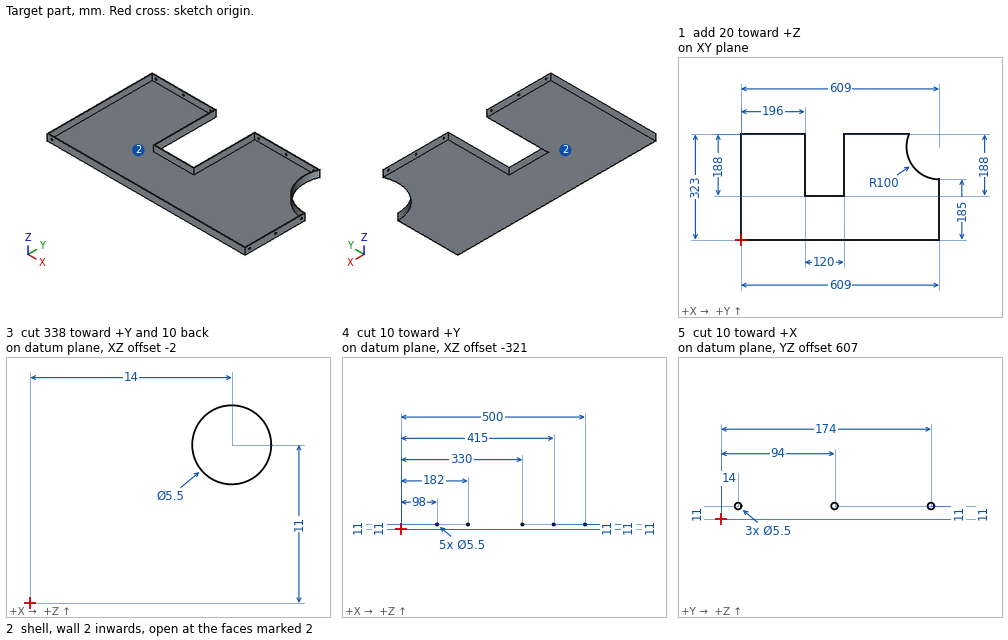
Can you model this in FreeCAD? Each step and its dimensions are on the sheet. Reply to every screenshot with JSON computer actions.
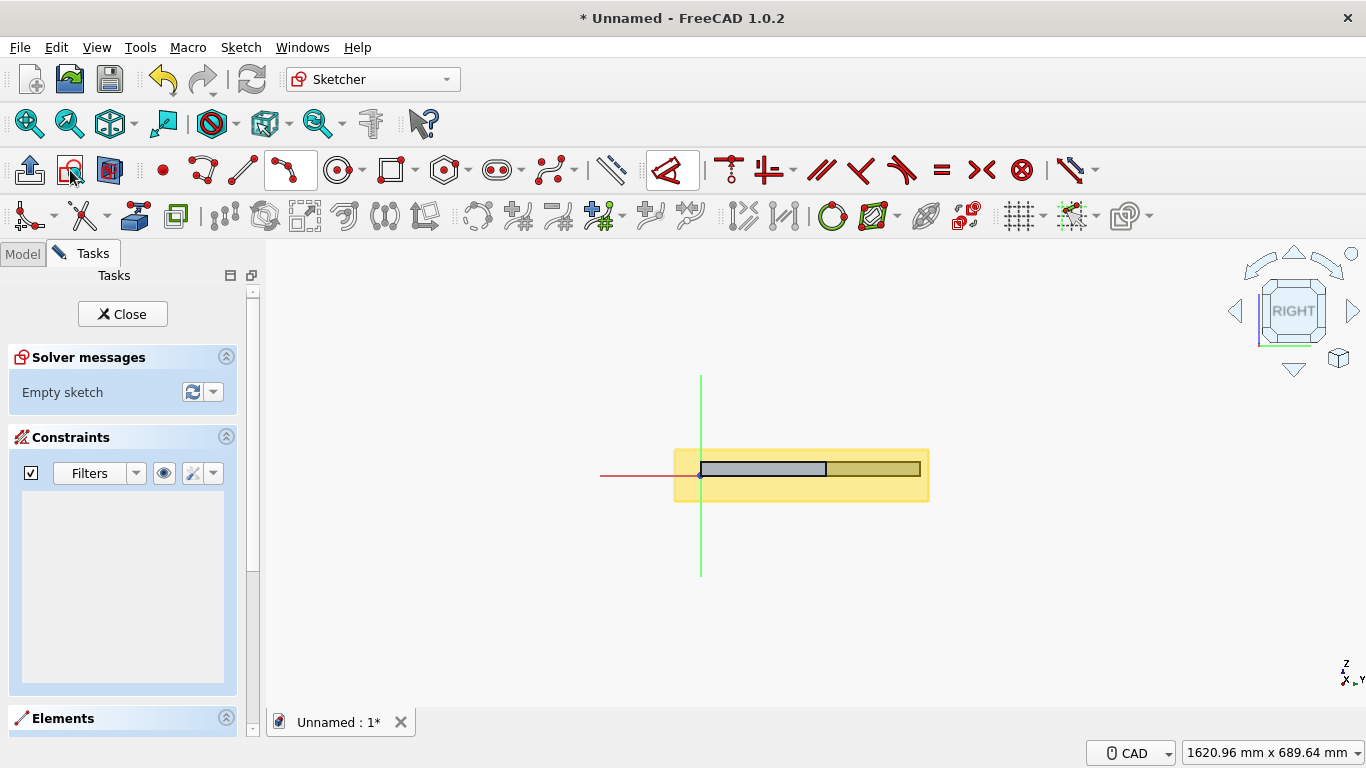
{"action": "key", "text": "q s"}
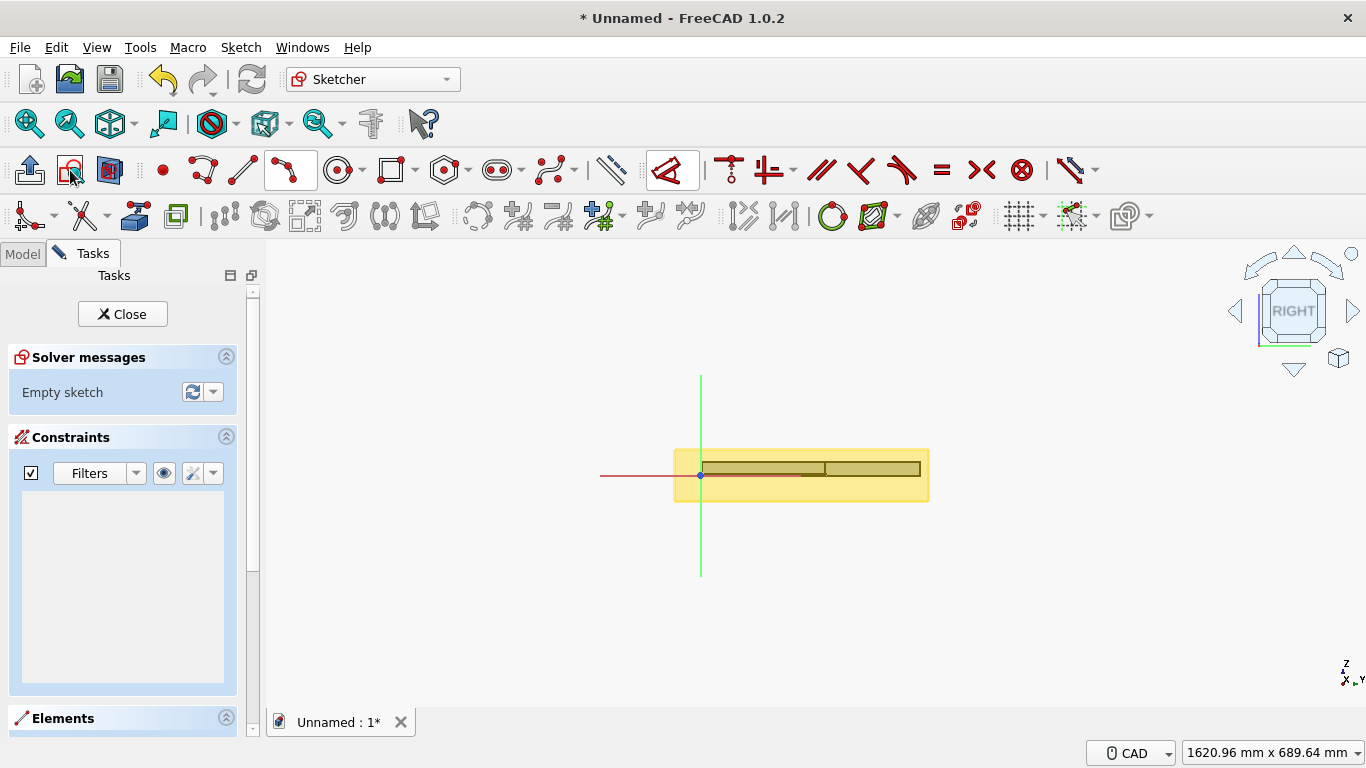
{"action": "scroll", "coordinate": [764, 470], "scroll_direction": "up", "scroll_amount": 8}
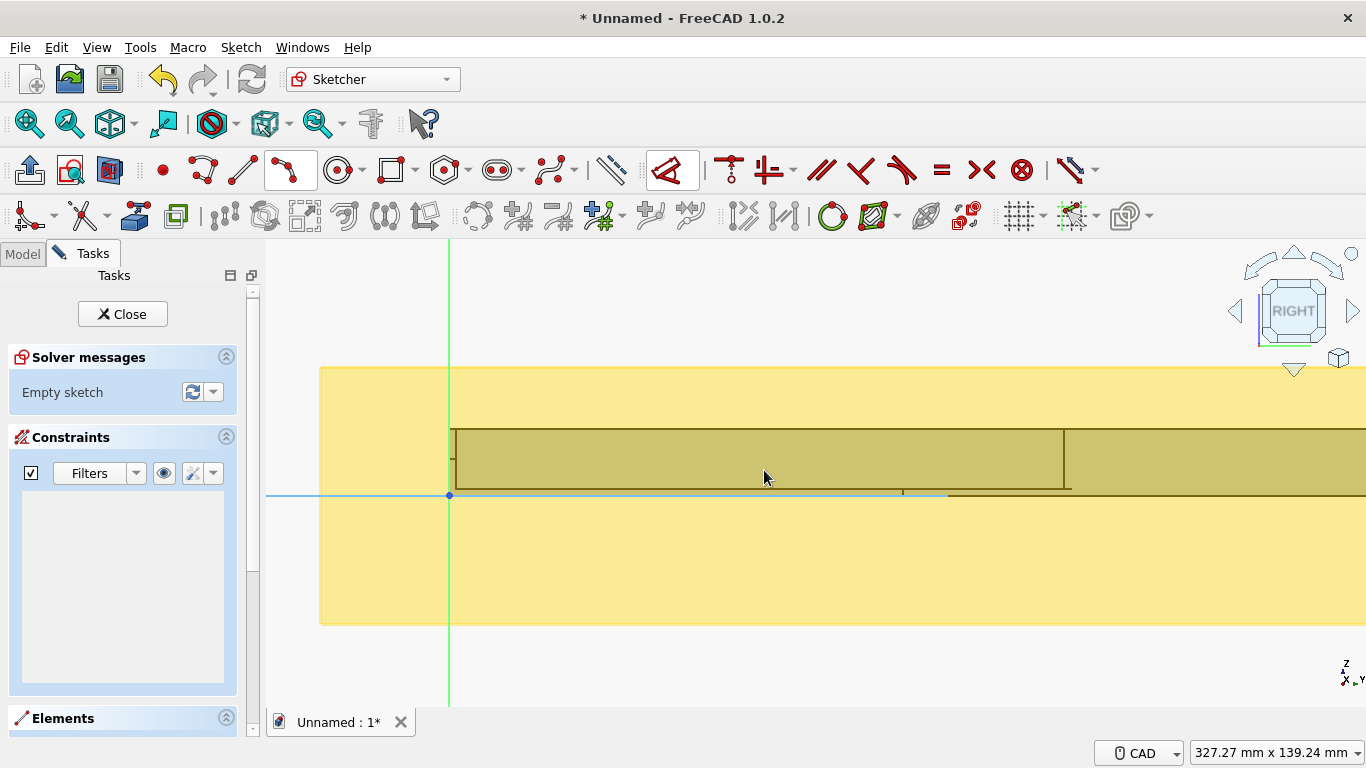
{"action": "key", "text": "g c"}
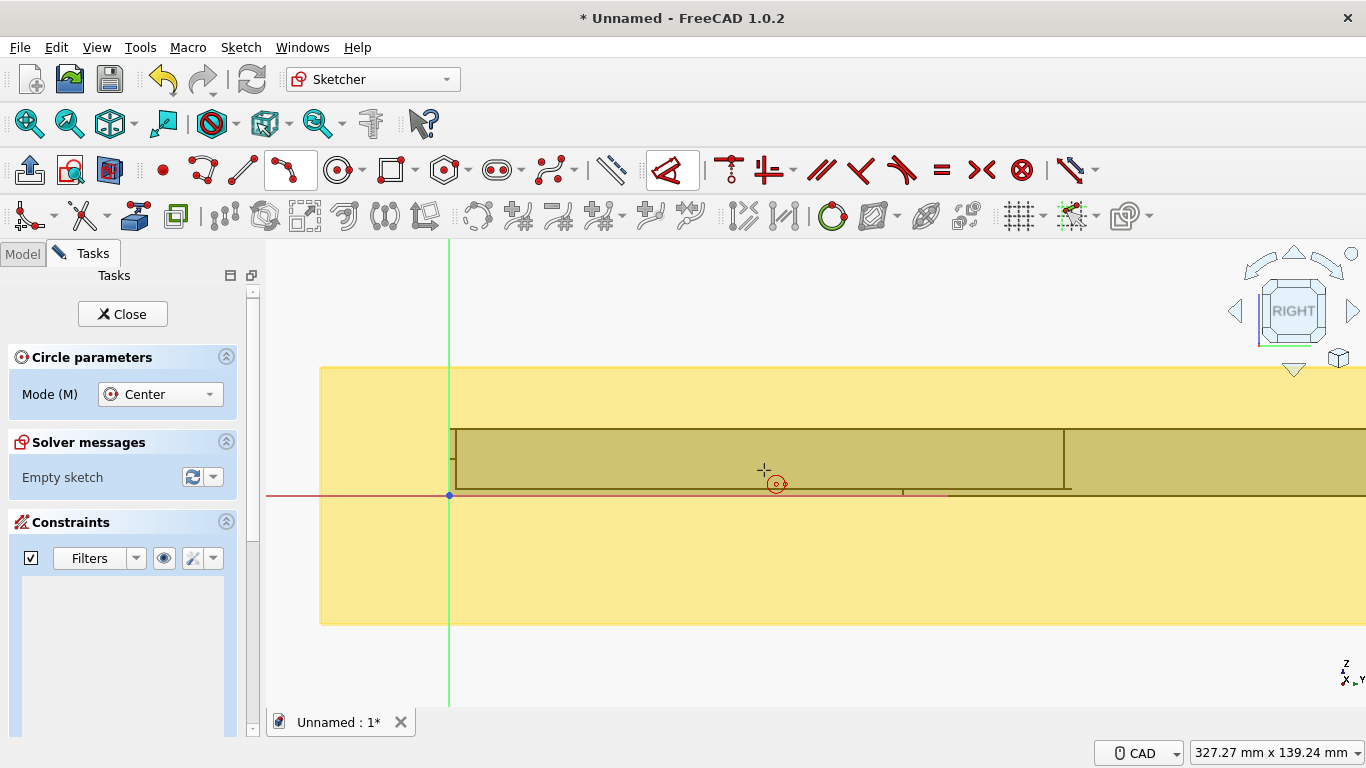
{"action": "scroll", "coordinate": [496, 459], "scroll_direction": "up", "scroll_amount": 5}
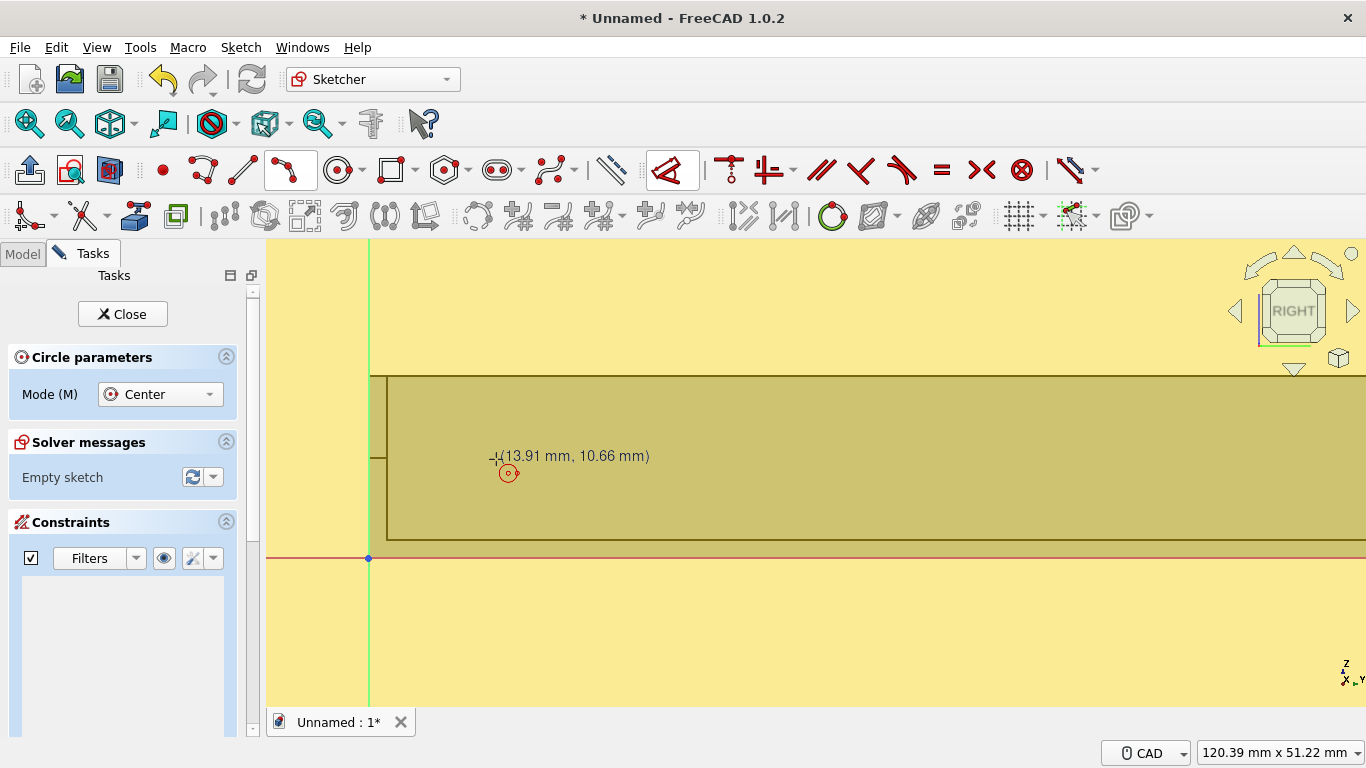
{"action": "left_click", "coordinate": [496, 458]}
{"action": "left_click", "coordinate": [514, 440]}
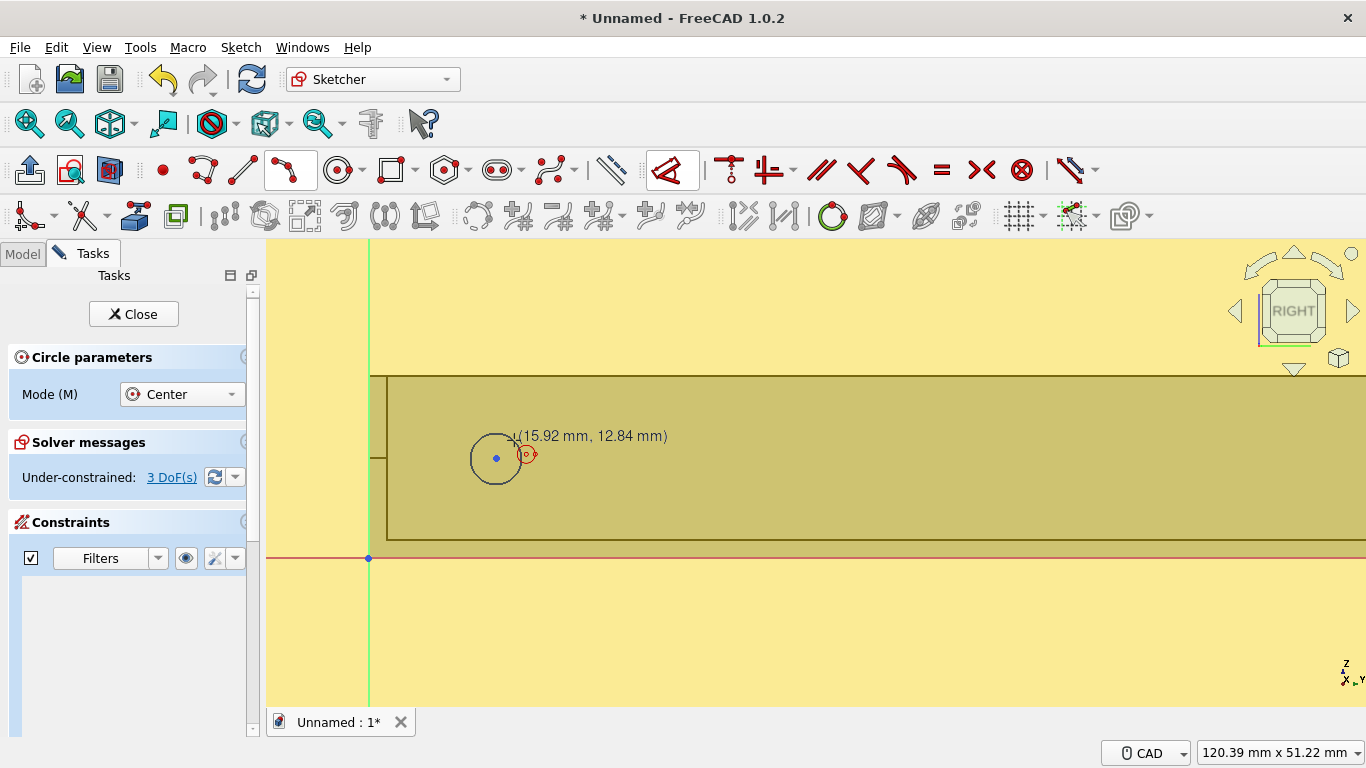
{"action": "scroll", "coordinate": [498, 460], "scroll_direction": "down", "scroll_amount": 5}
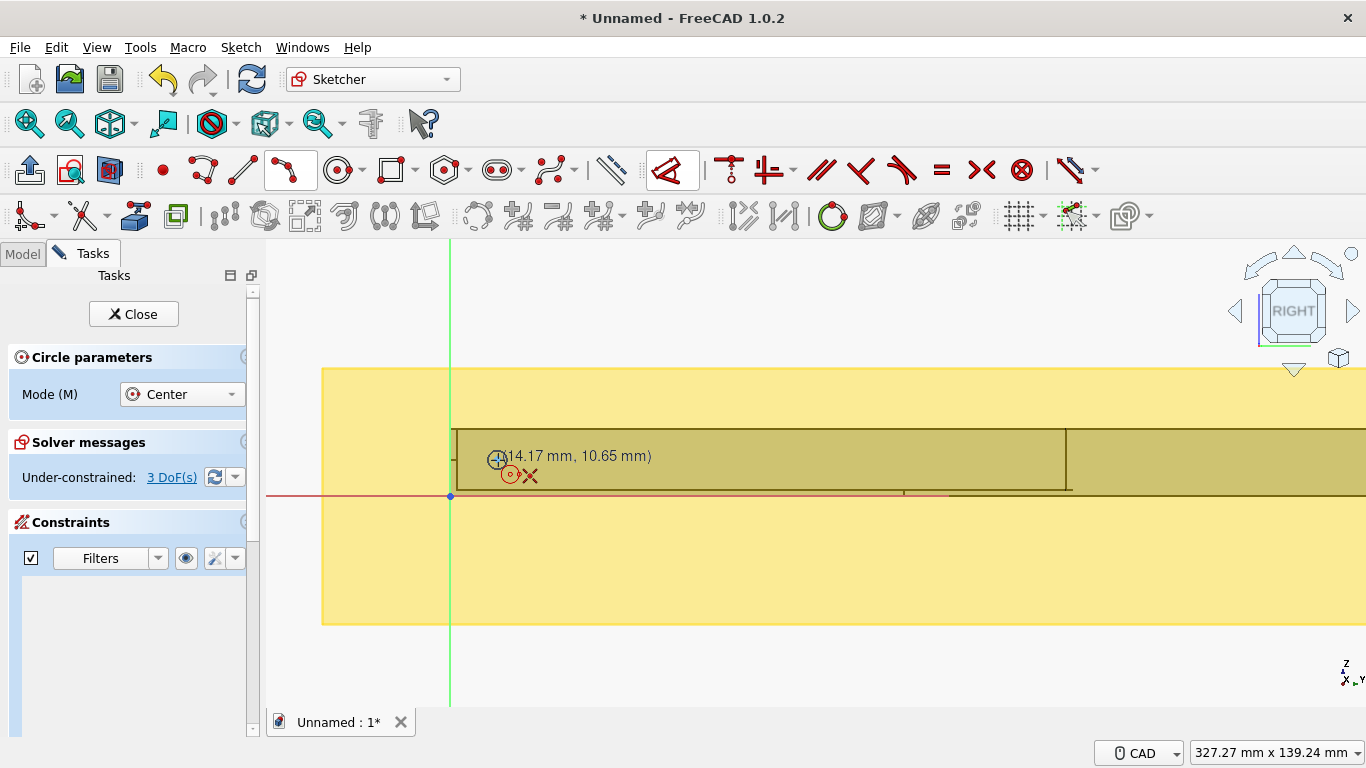
{"action": "scroll", "coordinate": [766, 460], "scroll_direction": "up", "scroll_amount": 5}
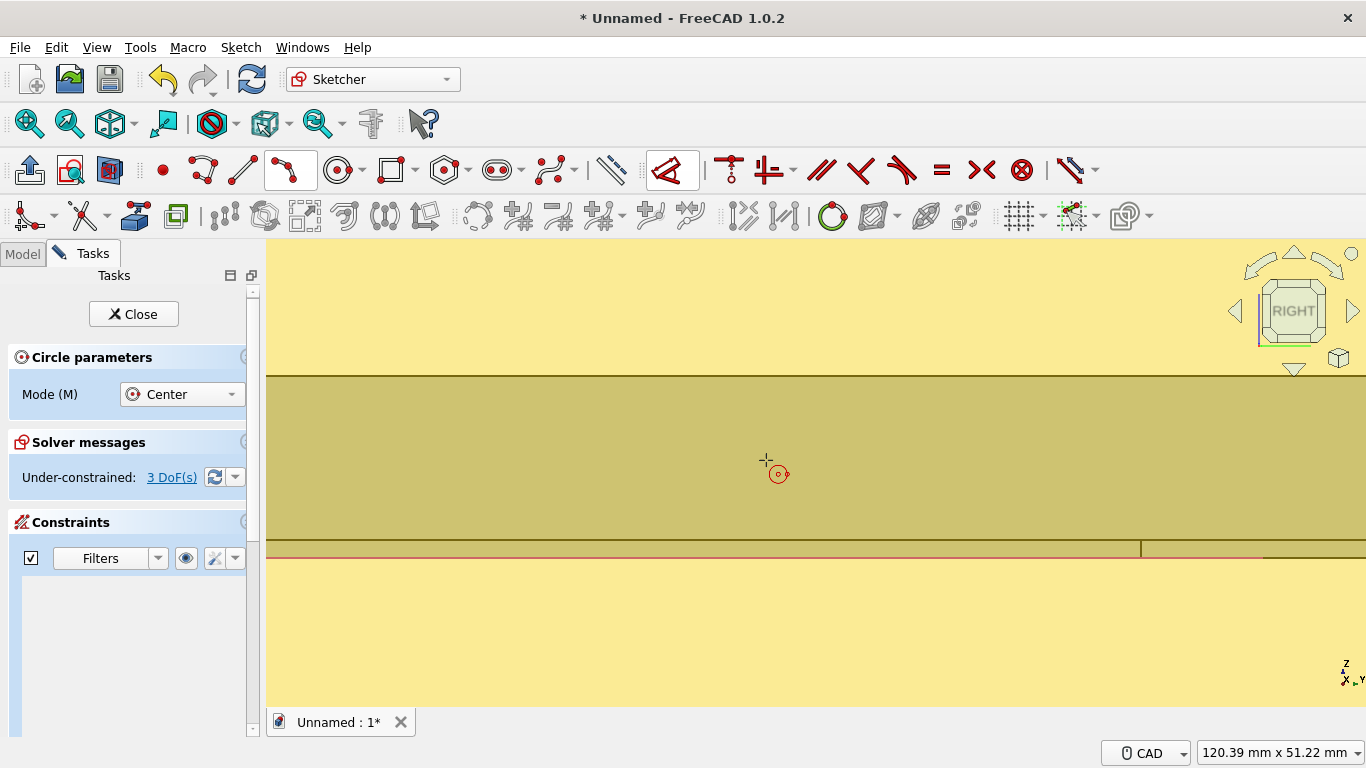
{"action": "left_click", "coordinate": [766, 458]}
{"action": "left_click", "coordinate": [784, 440]}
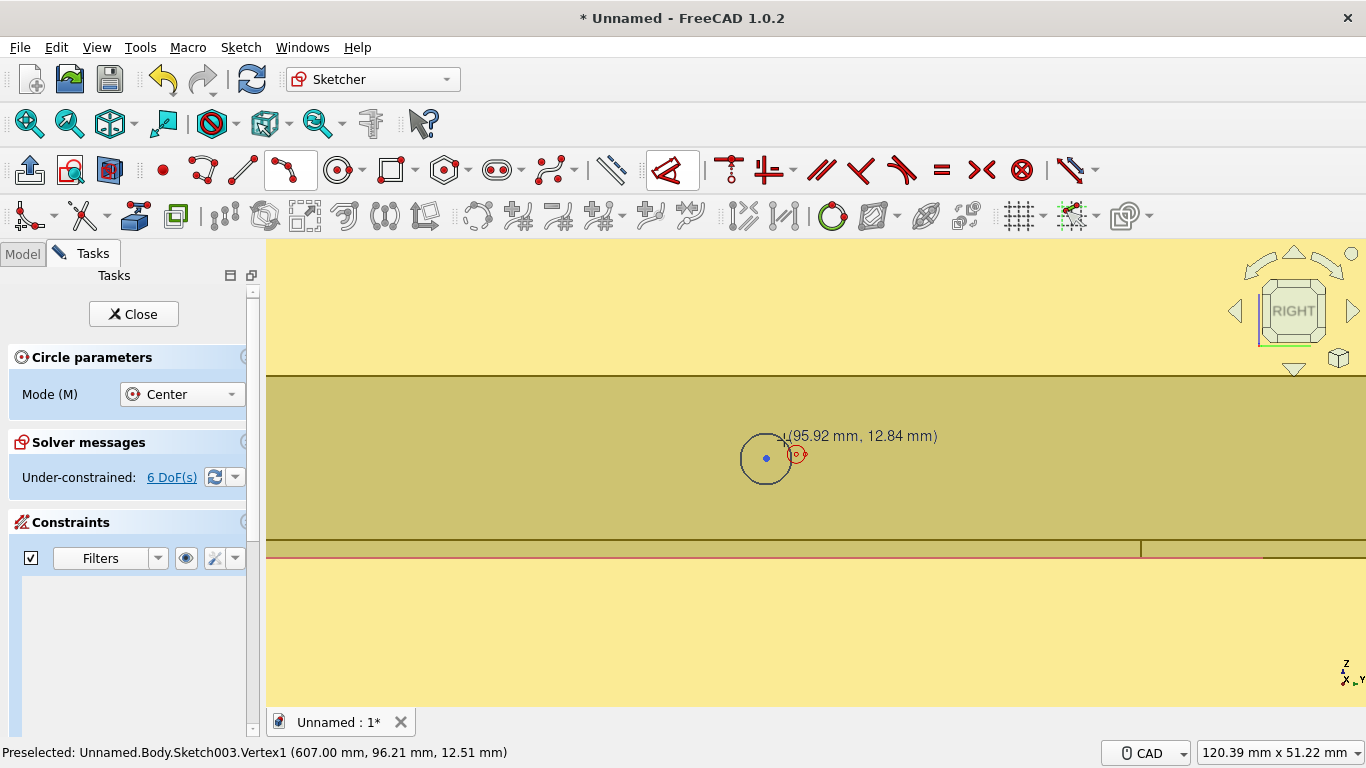
{"action": "scroll", "coordinate": [766, 460], "scroll_direction": "down", "scroll_amount": 5}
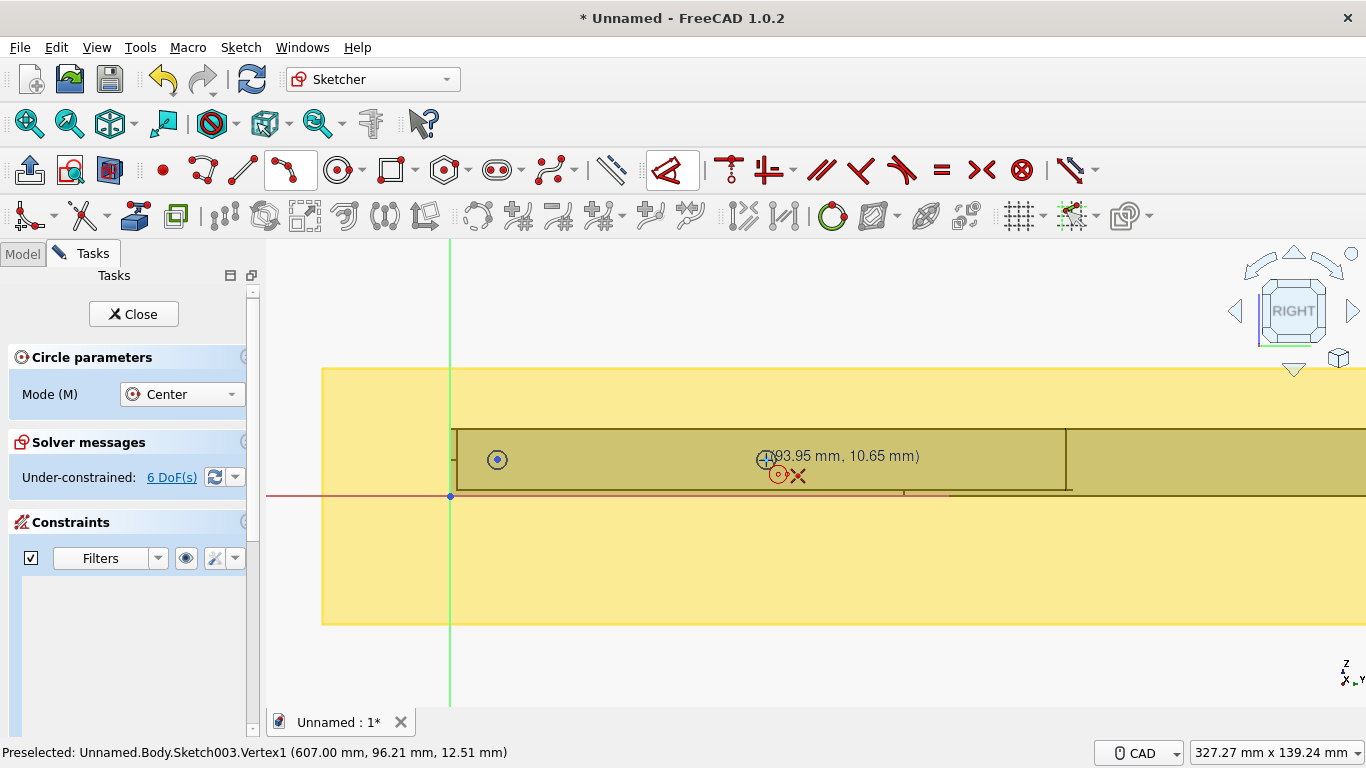
{"action": "scroll", "coordinate": [1035, 460], "scroll_direction": "up", "scroll_amount": 5}